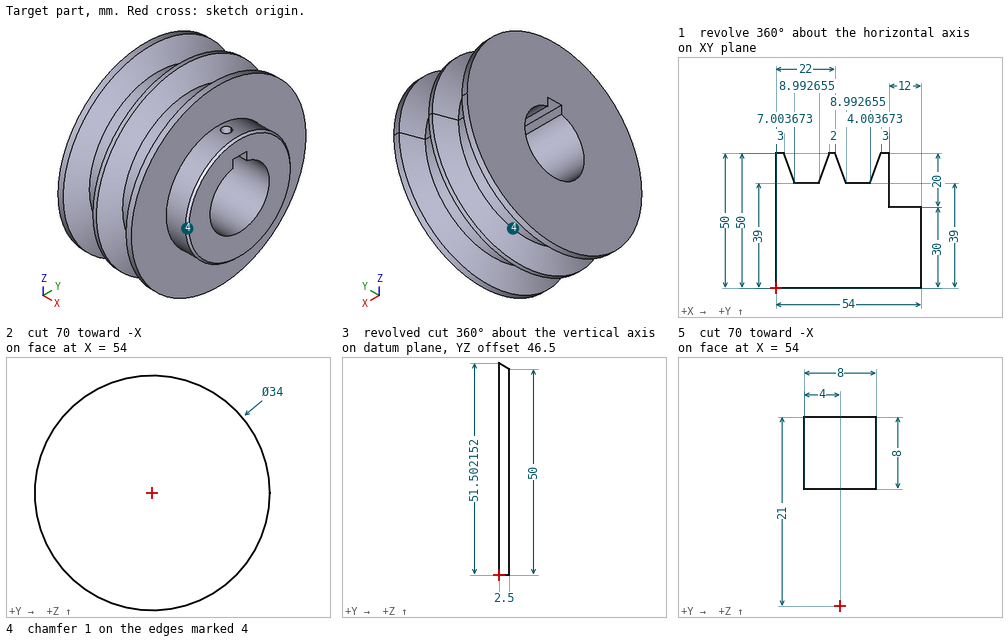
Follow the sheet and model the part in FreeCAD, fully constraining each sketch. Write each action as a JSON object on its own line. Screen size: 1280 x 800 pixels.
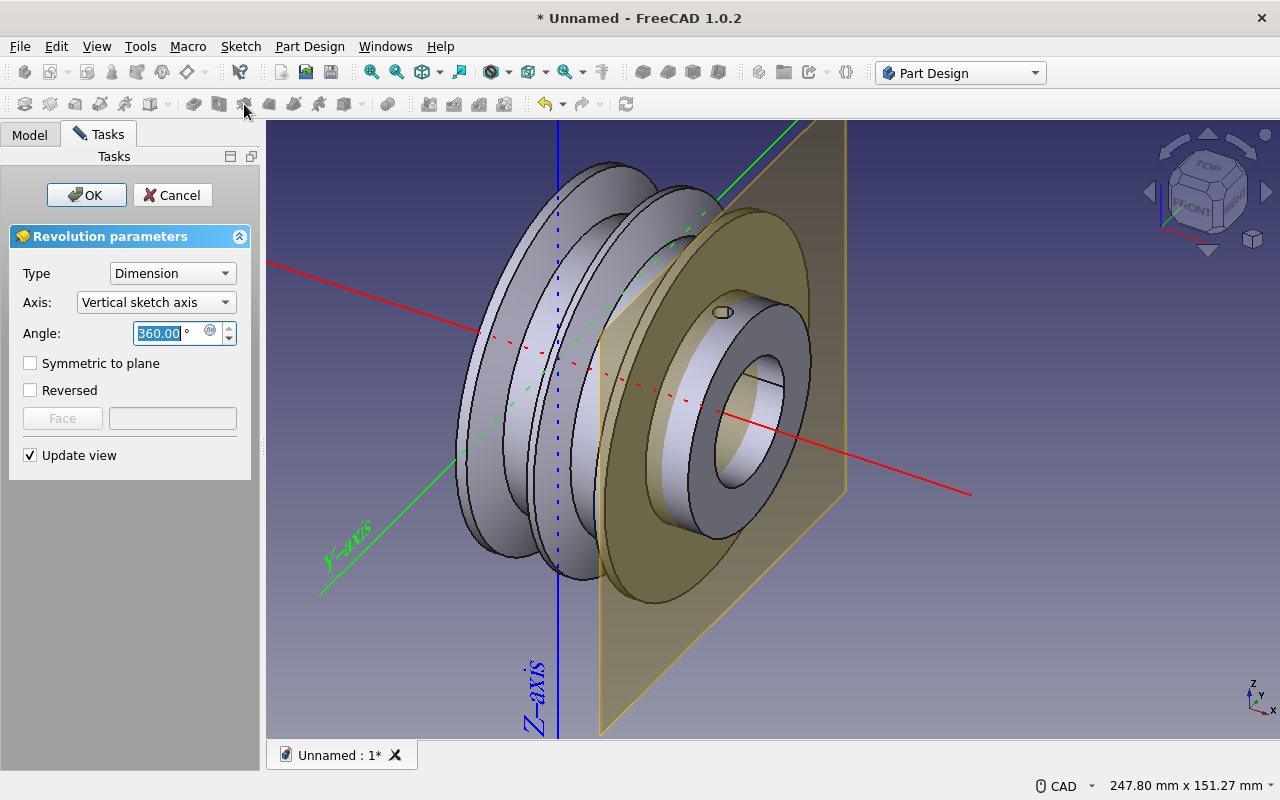
{"action": "left_click", "coordinate": [87, 195]}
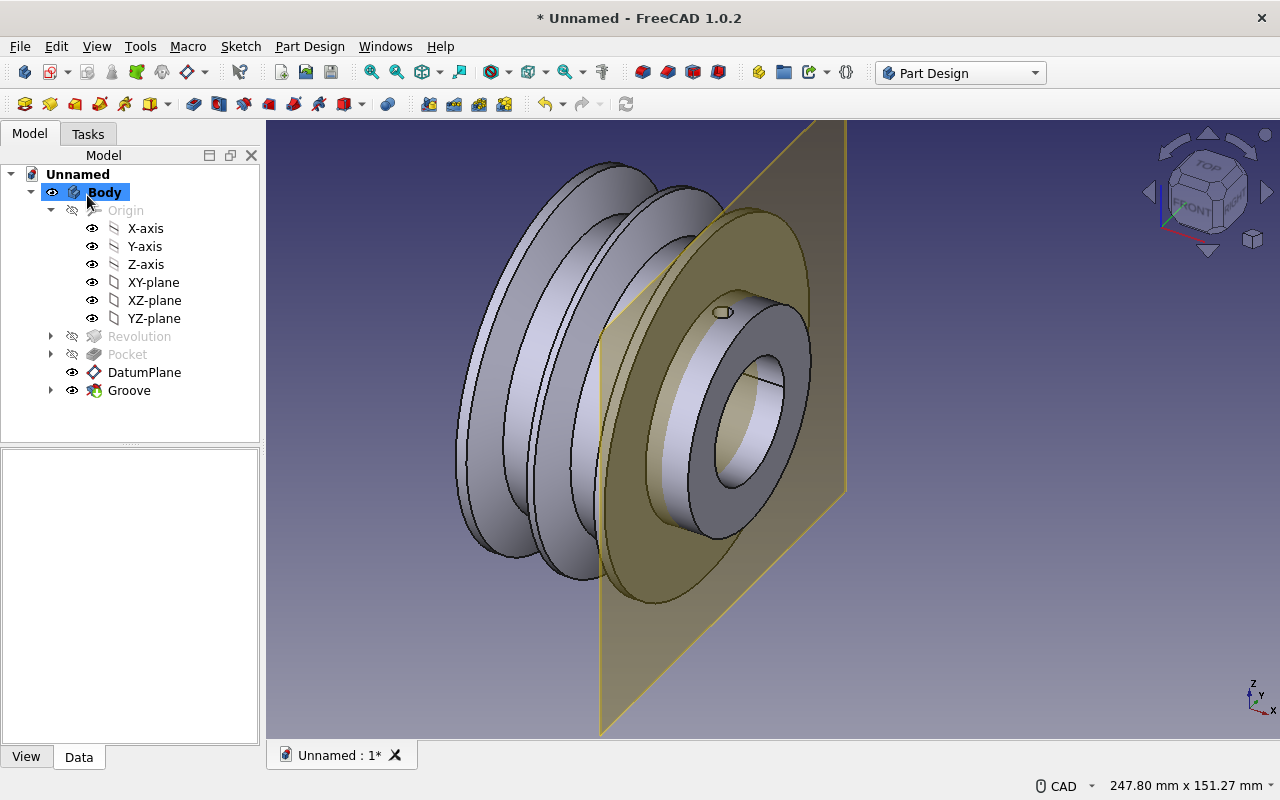
{"action": "left_click", "coordinate": [117, 372]}
{"action": "key", "text": "space"}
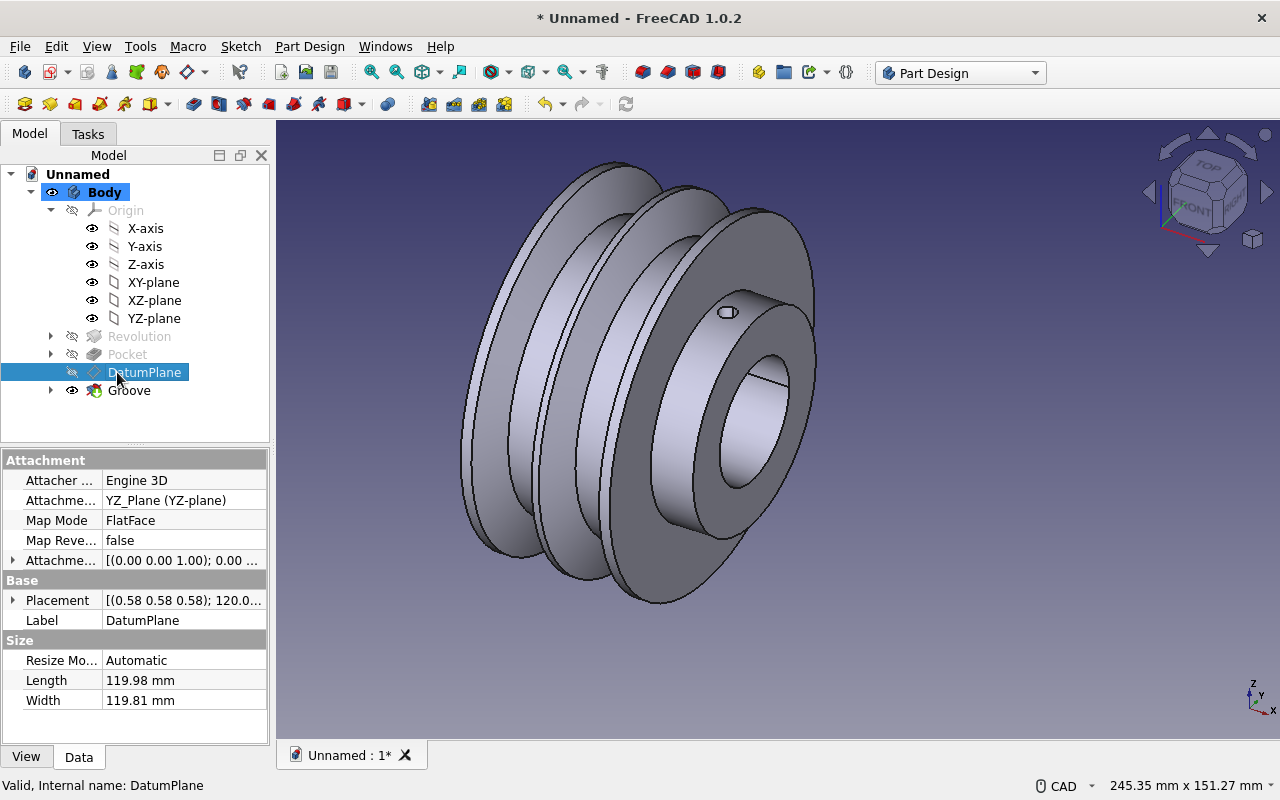
{"action": "key", "text": "v f"}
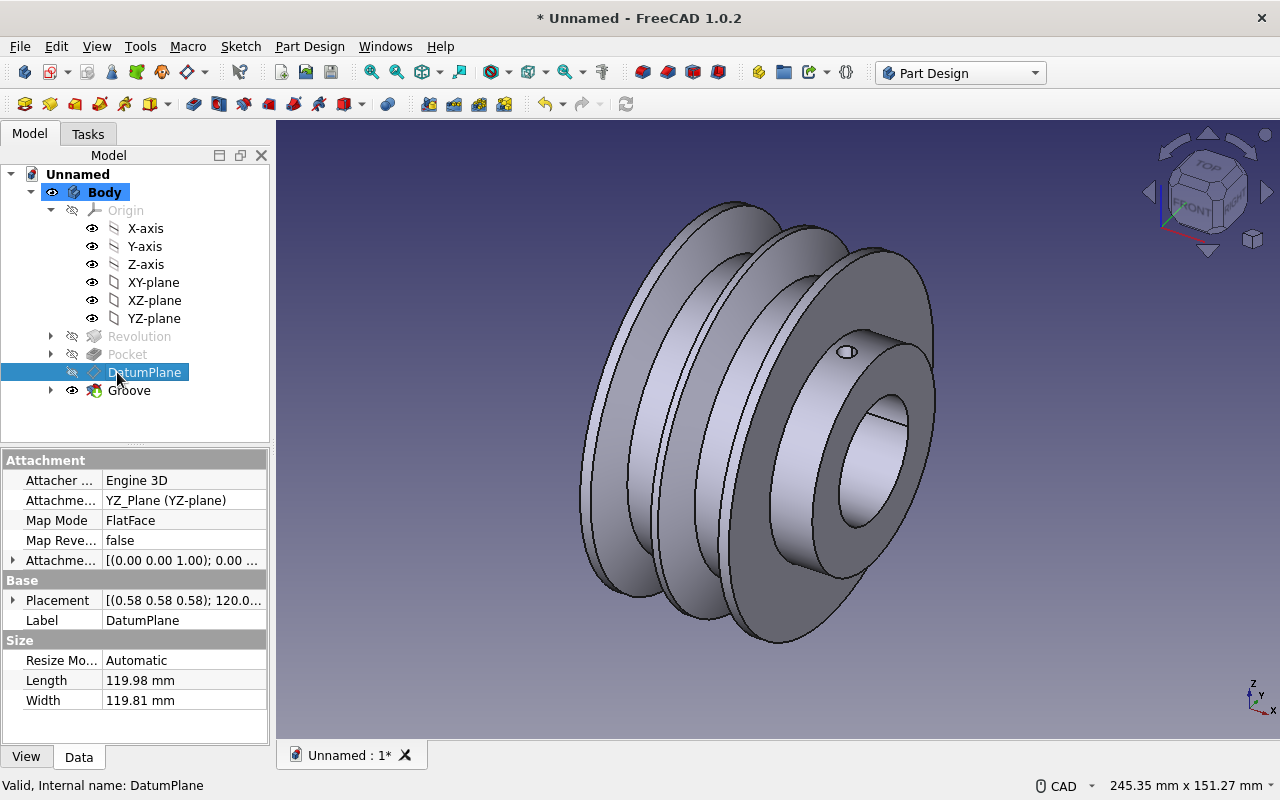
{"action": "left_click", "coordinate": [812, 521]}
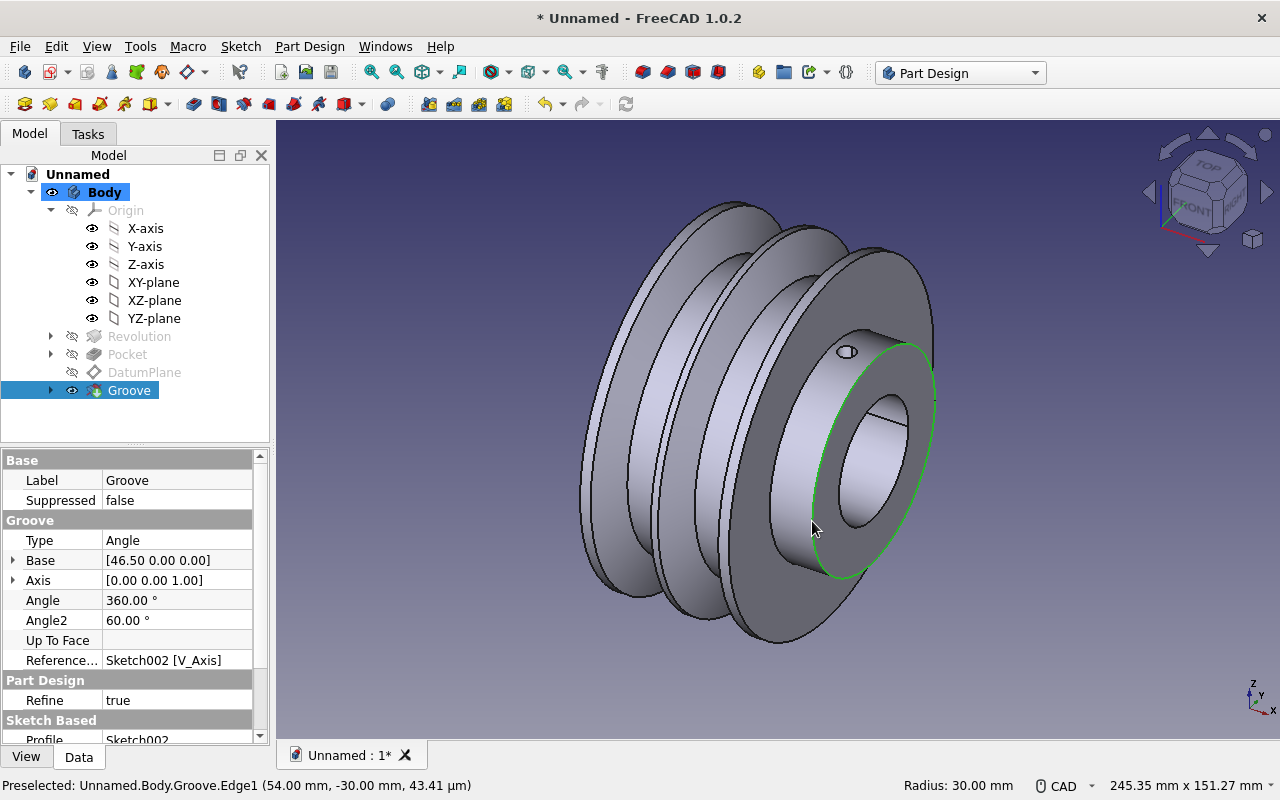
{"action": "left_click", "coordinate": [668, 72]}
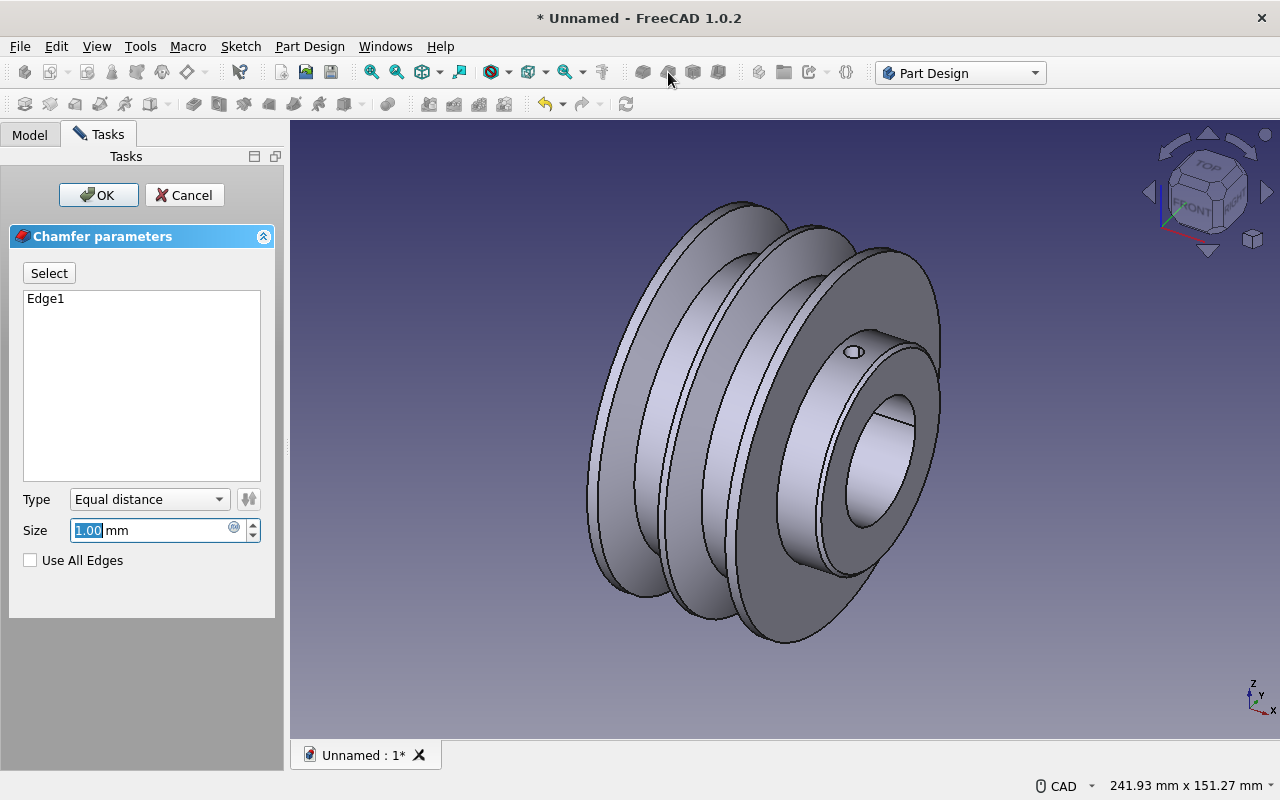
{"action": "type", "text": "1"}
{"action": "key", "text": "Tab"}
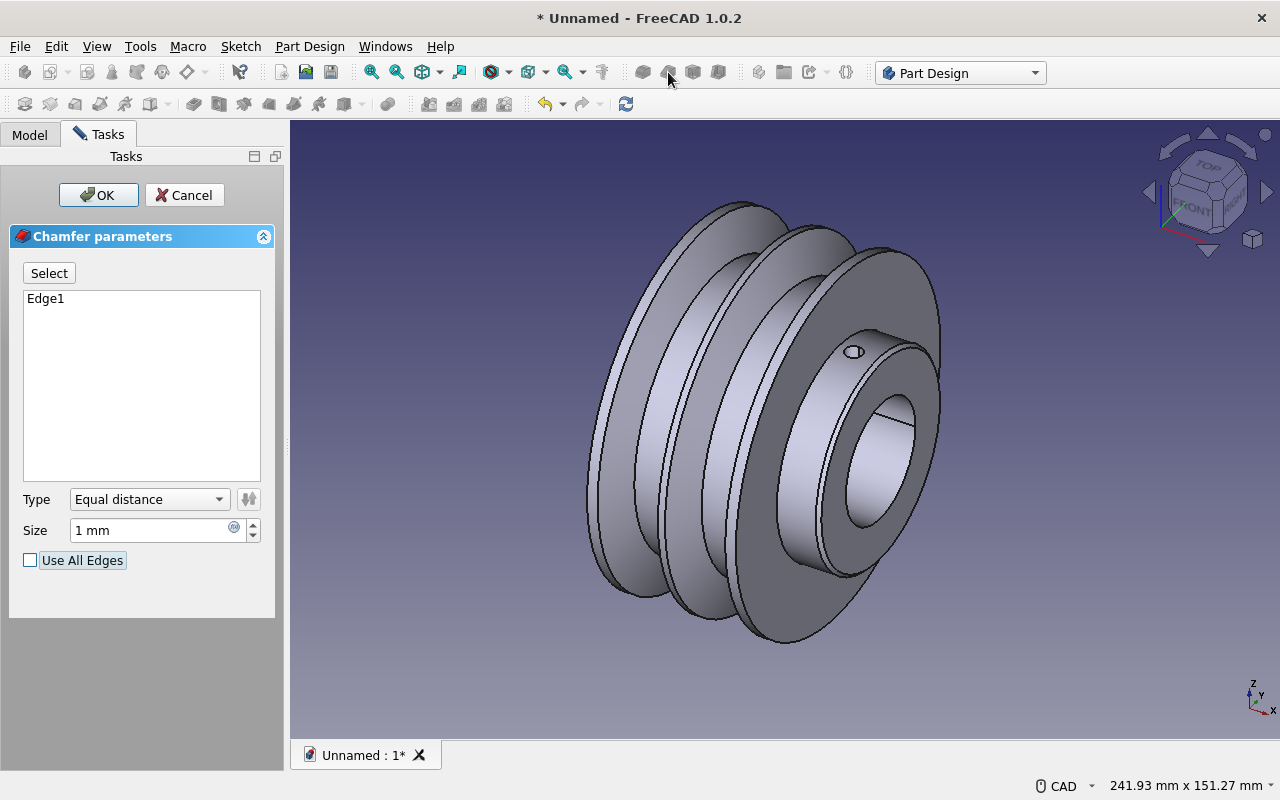
{"action": "left_click", "coordinate": [99, 195]}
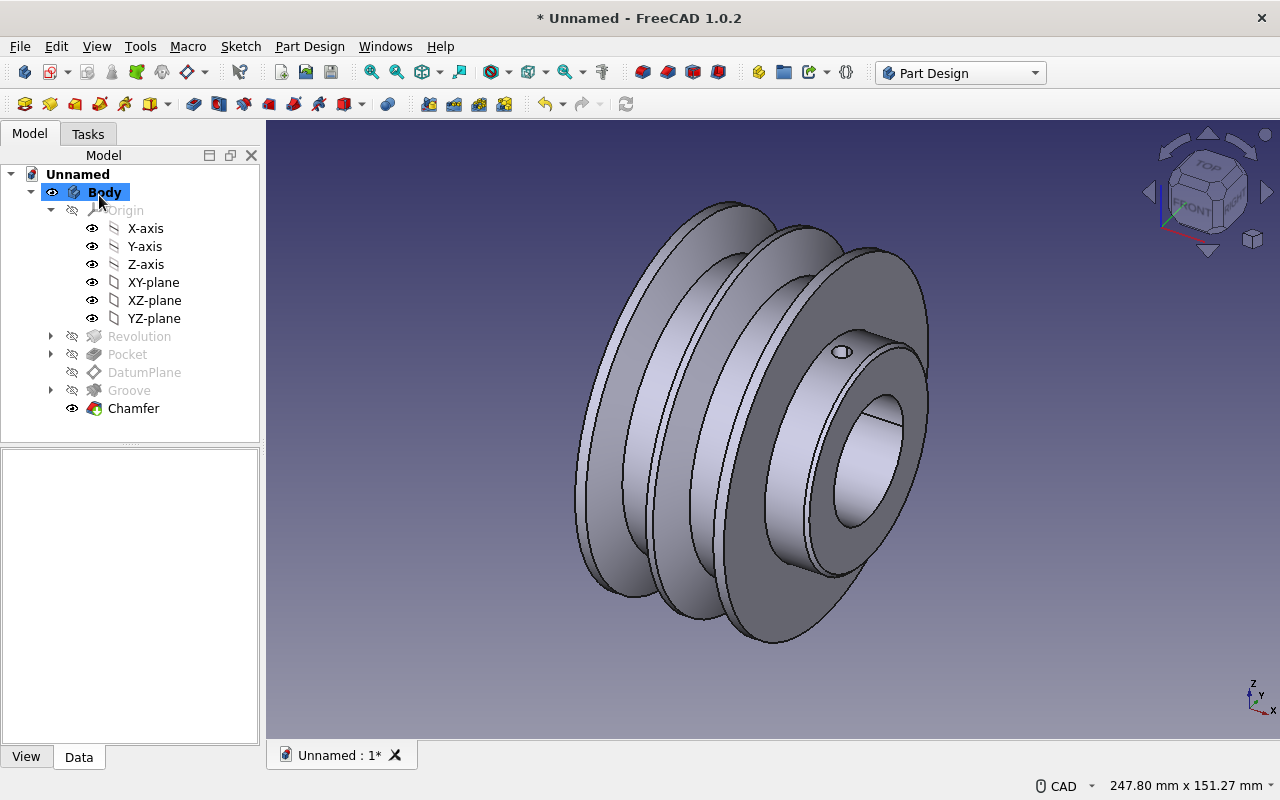
{"action": "left_click", "coordinate": [835, 549]}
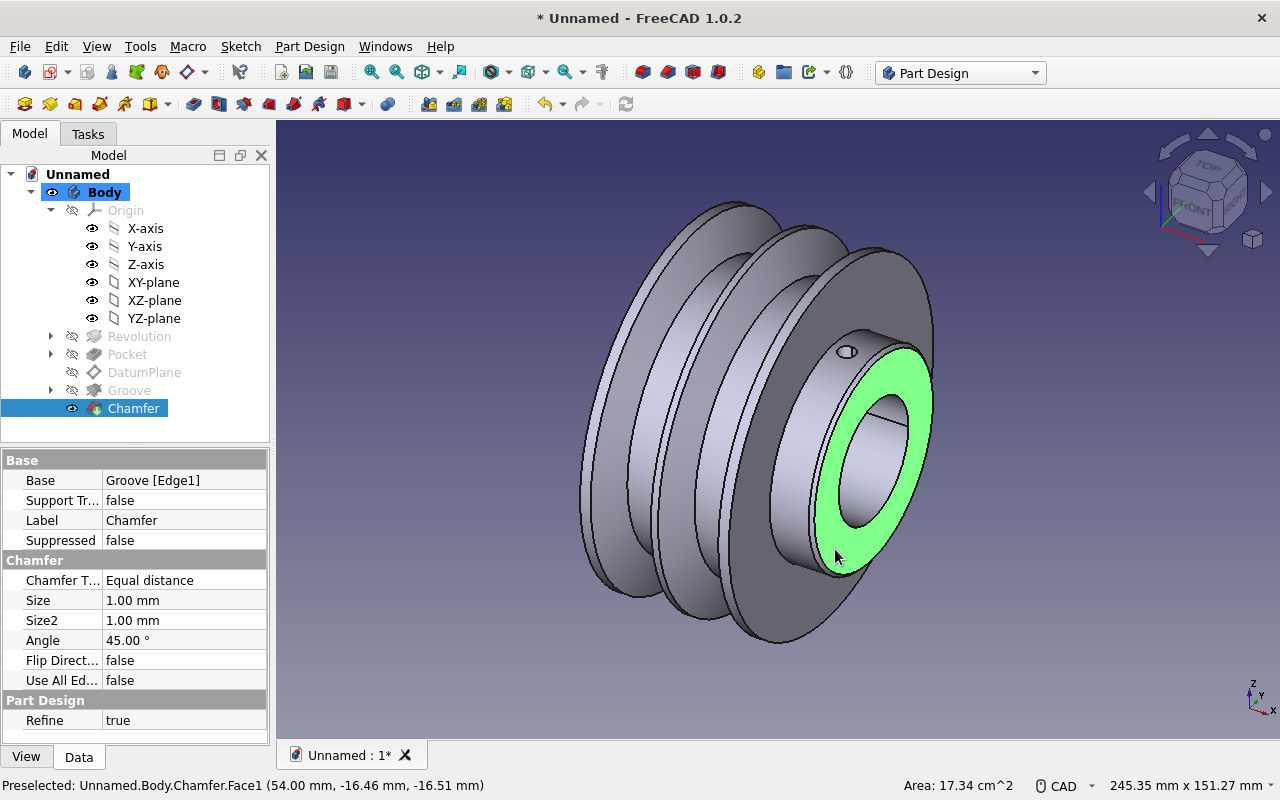
{"action": "left_click", "coordinate": [50, 72]}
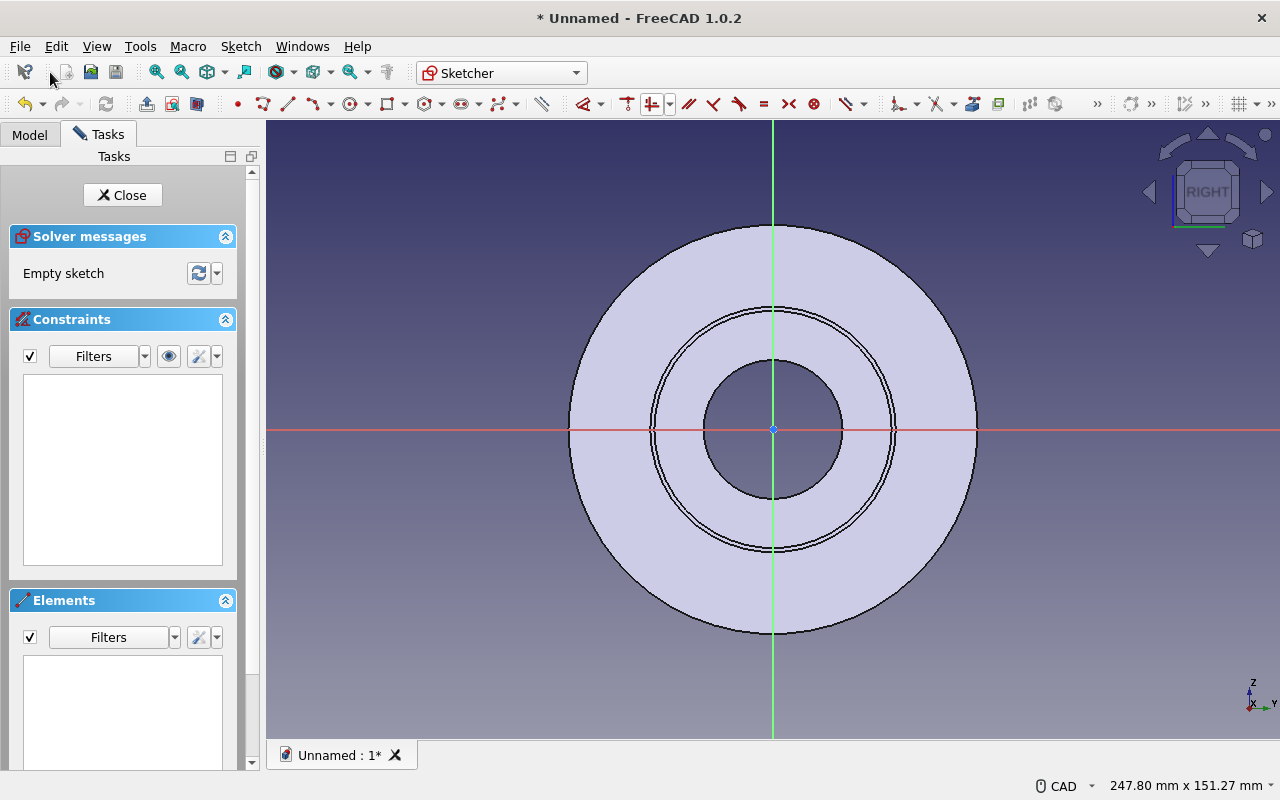
{"action": "scroll", "coordinate": [780, 353], "scroll_direction": "up", "scroll_amount": 12}